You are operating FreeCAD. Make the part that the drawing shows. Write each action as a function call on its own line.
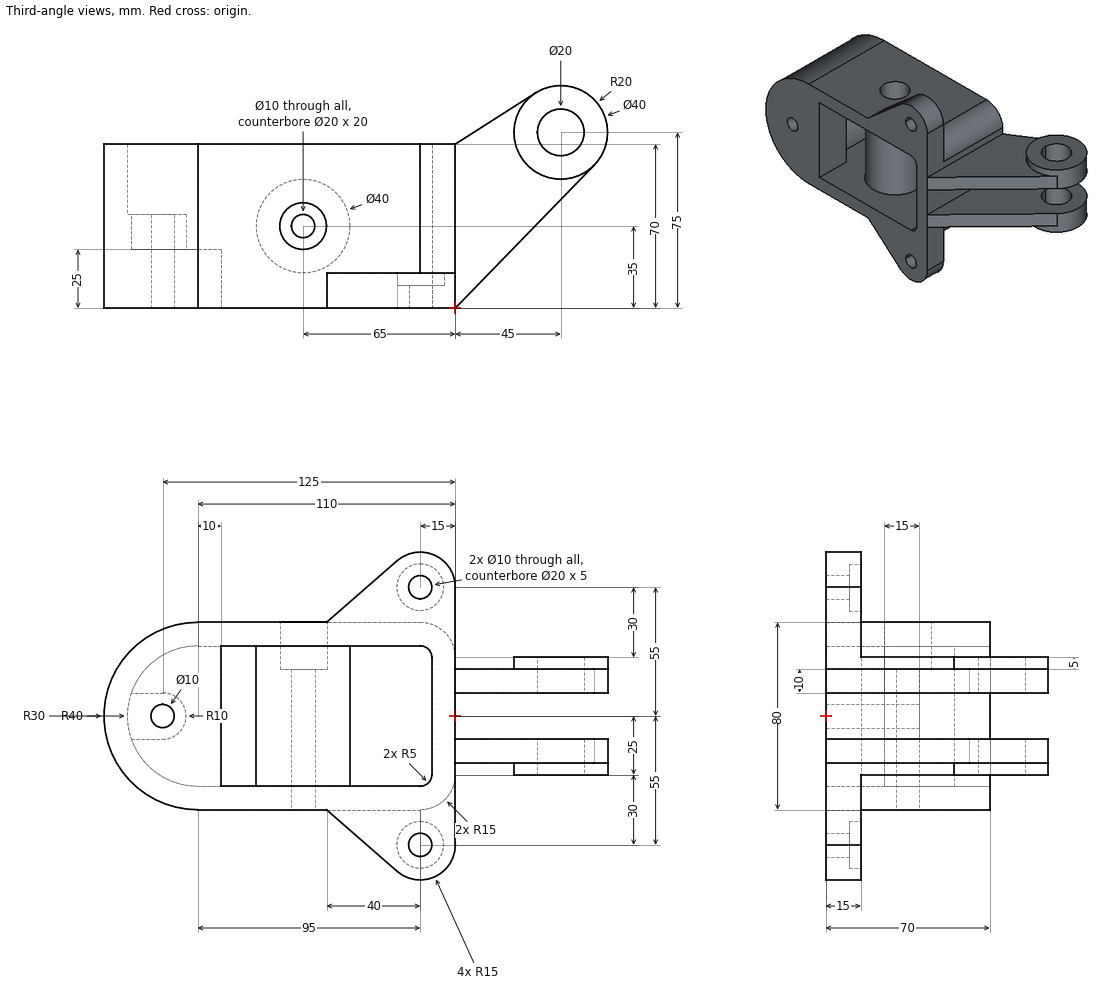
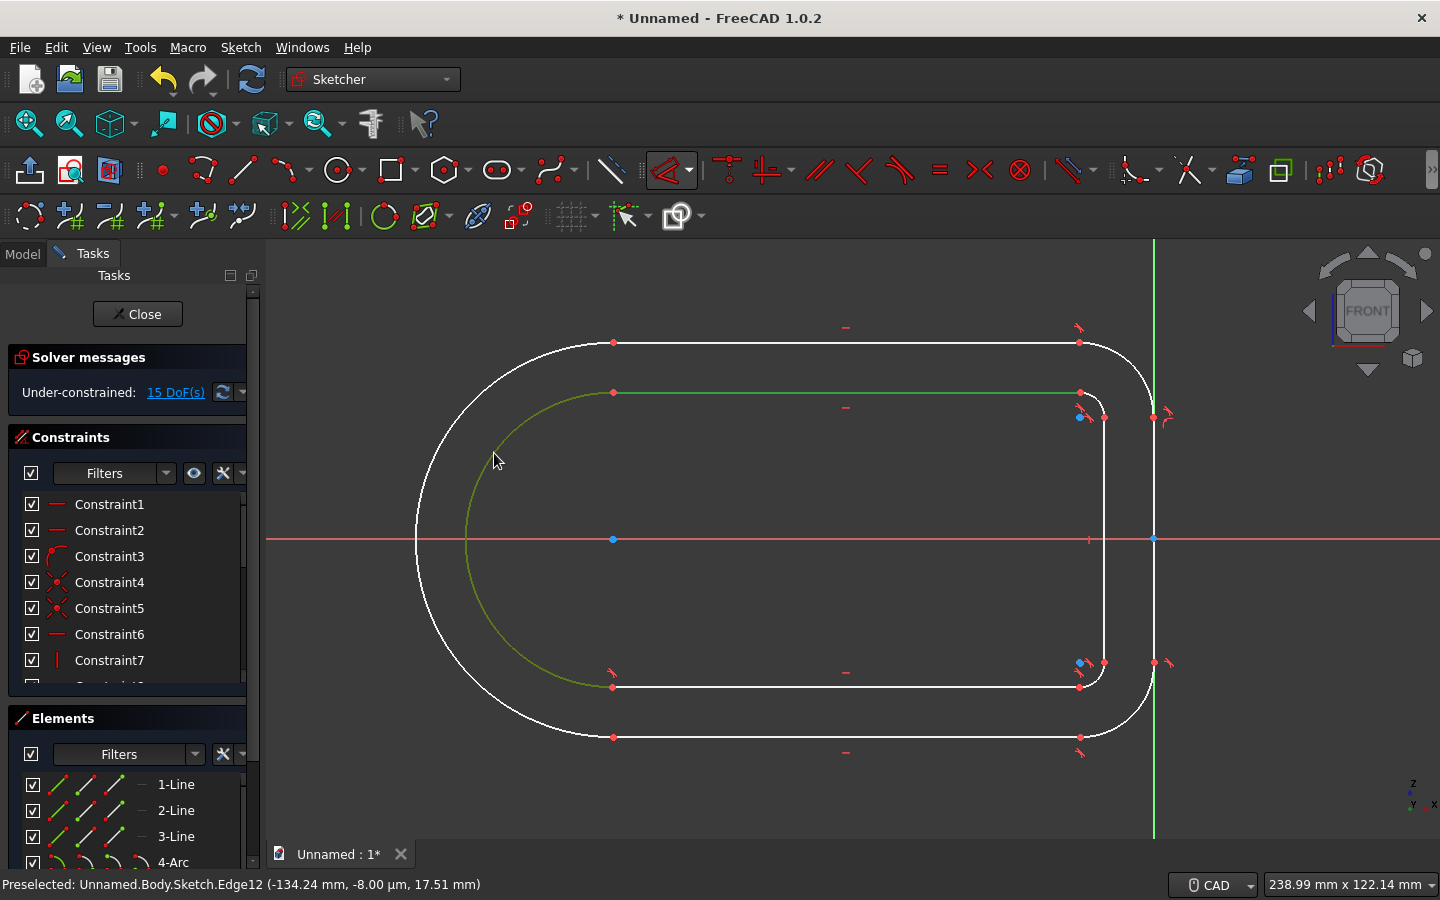
click(900, 170)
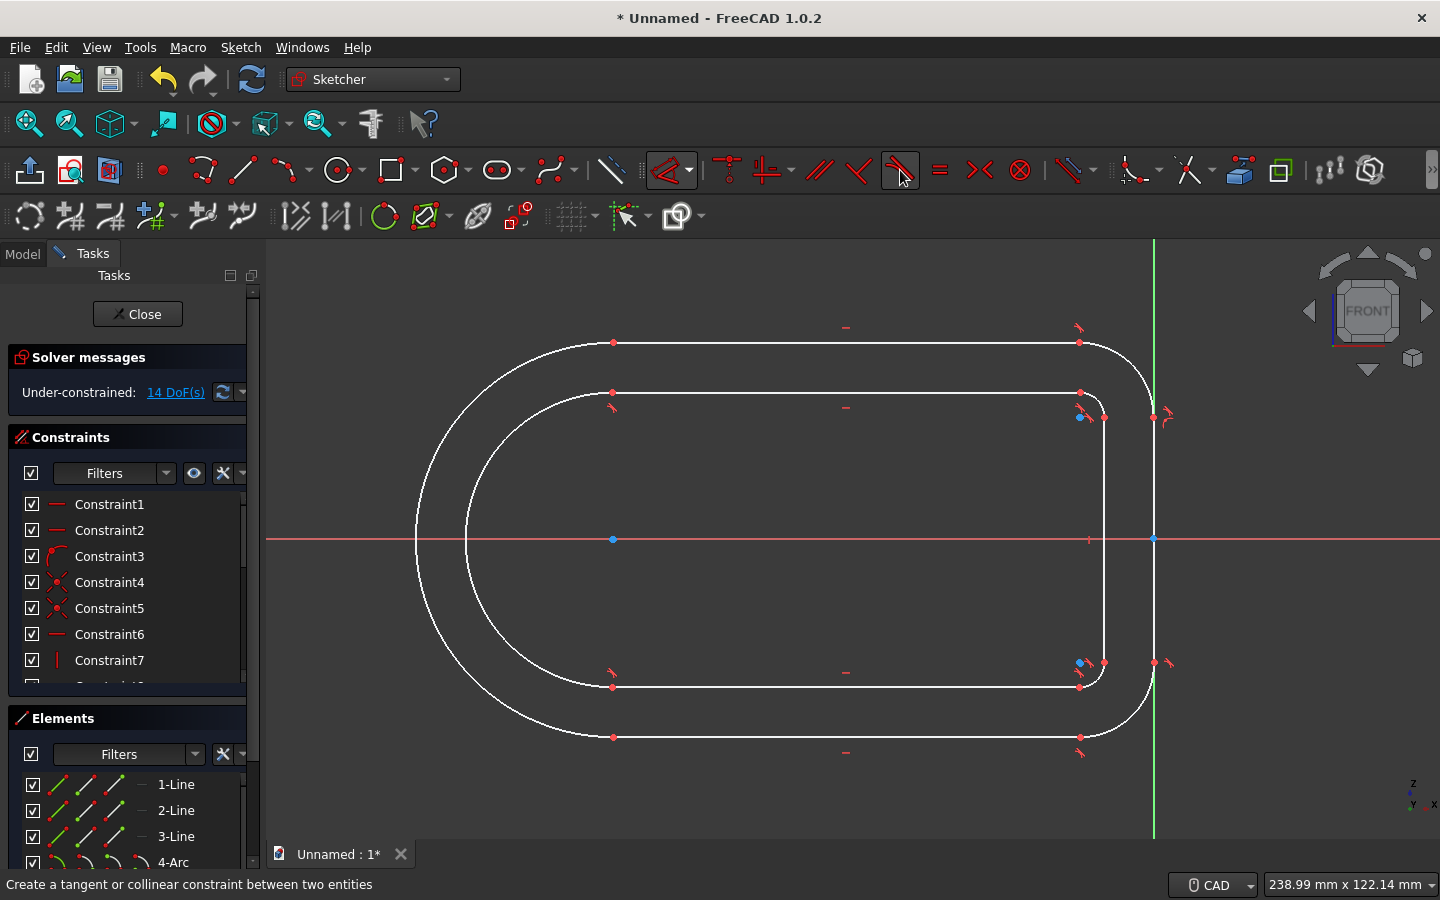
click(1154, 491)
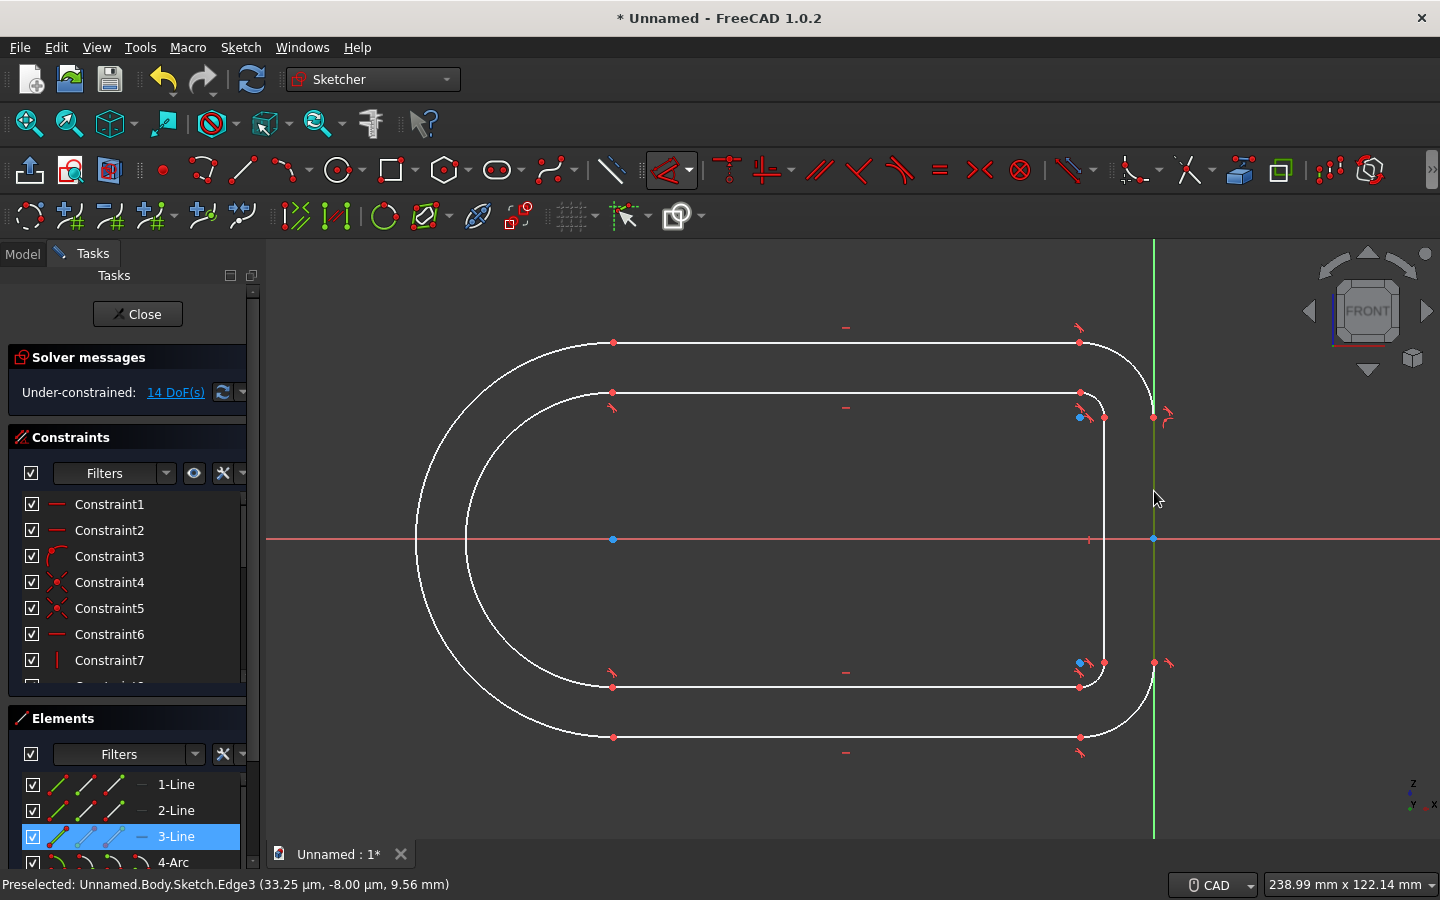
key(v)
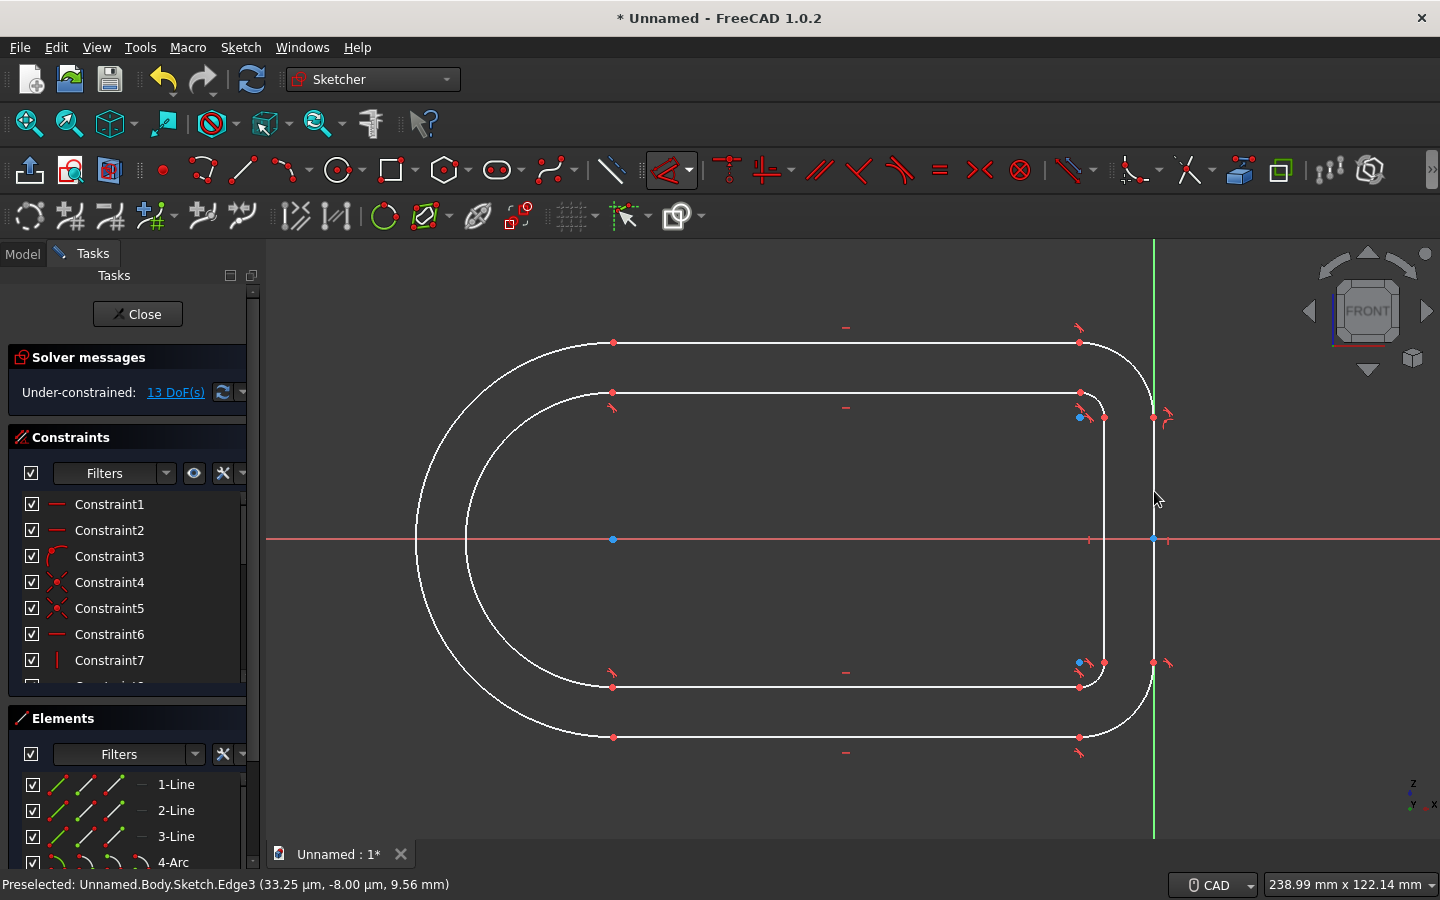
click(1113, 729)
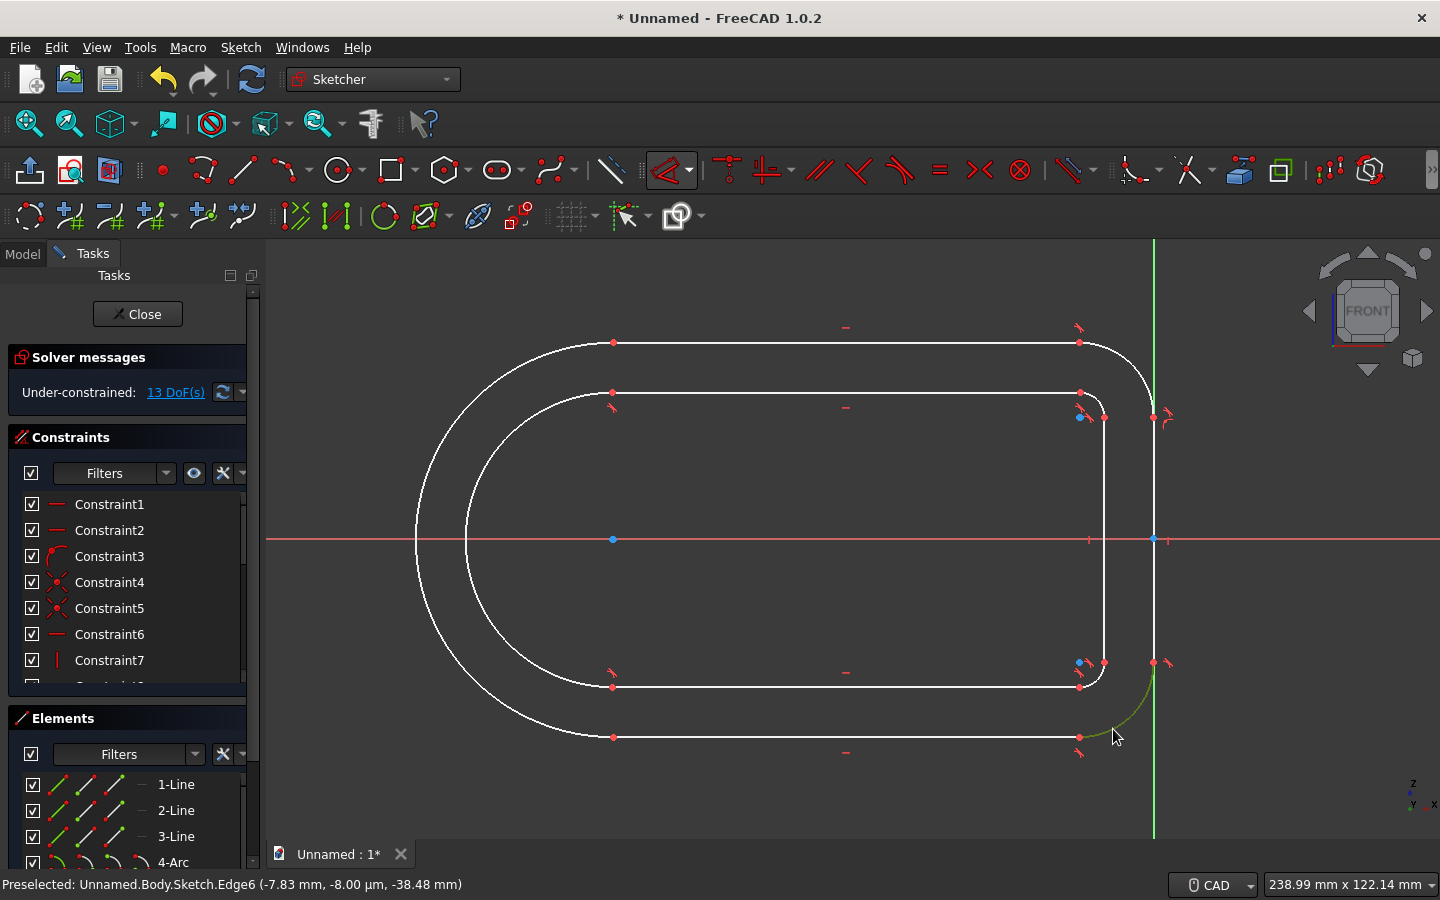
click(1091, 685)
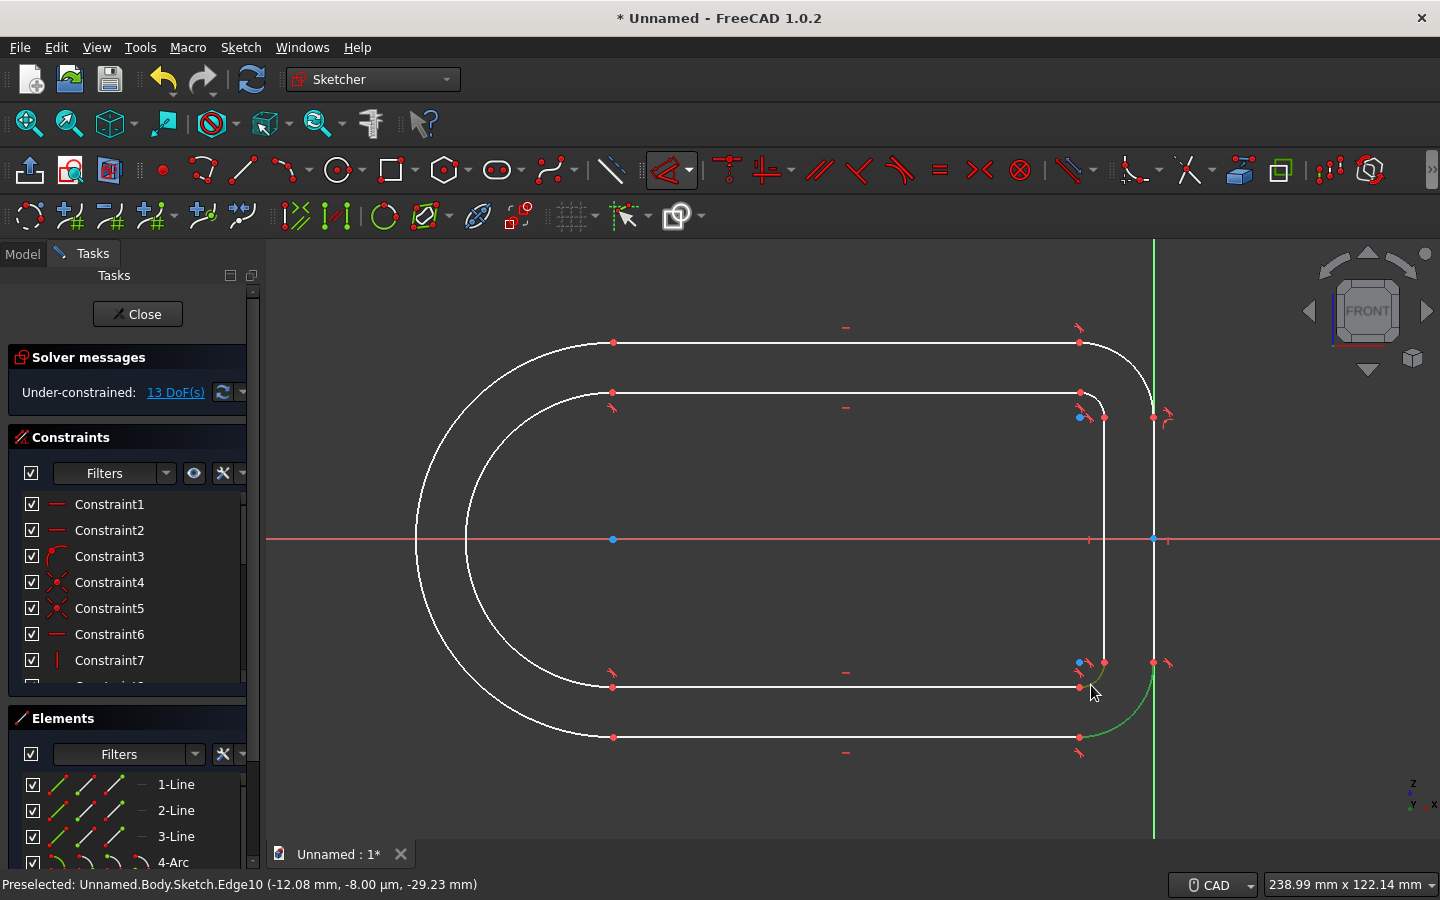
click(728, 170)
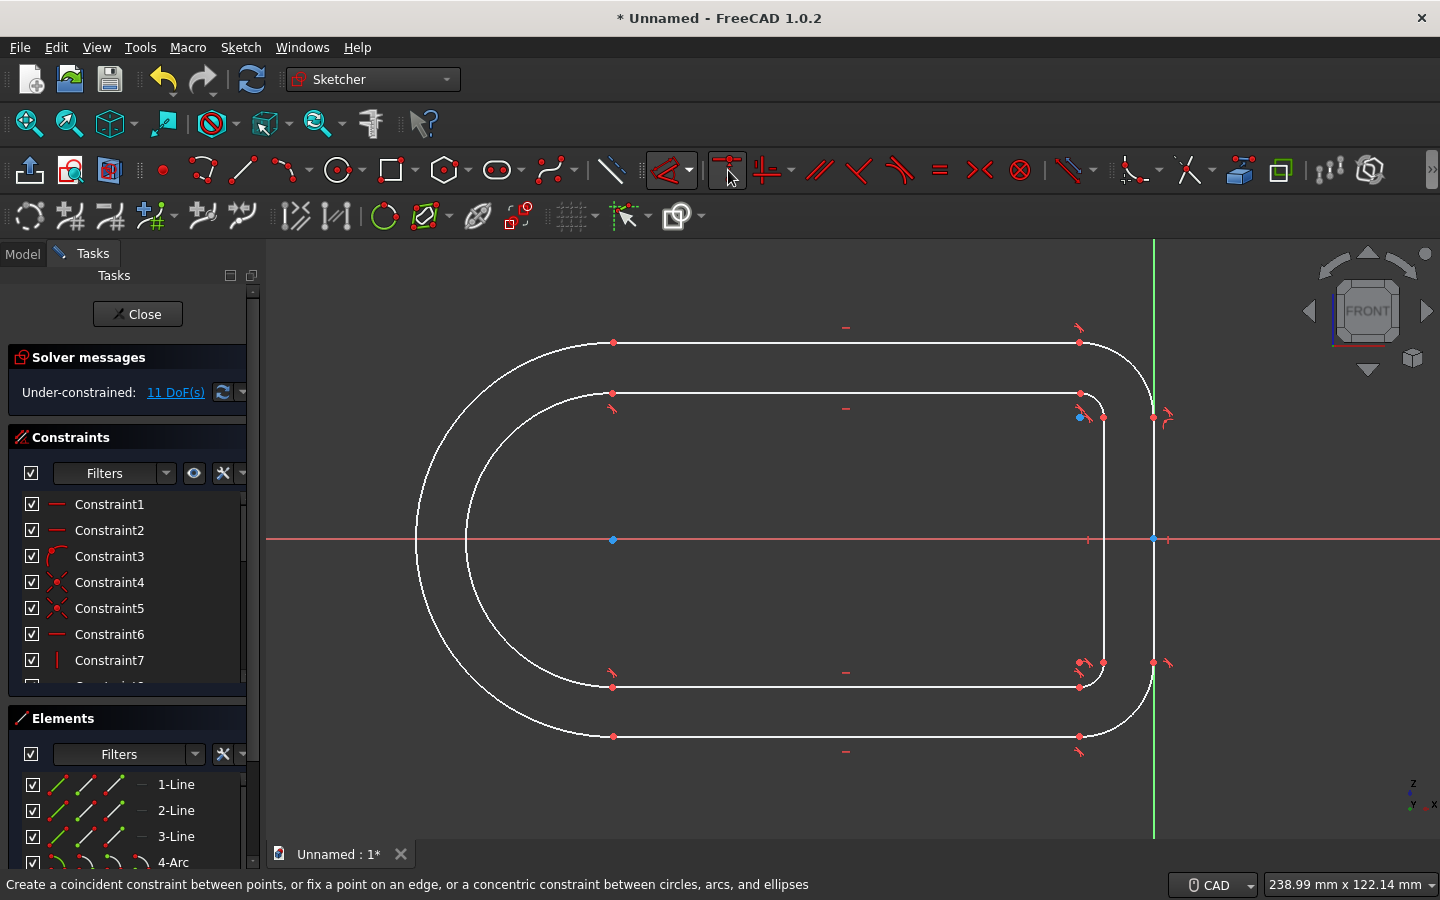
click(1113, 351)